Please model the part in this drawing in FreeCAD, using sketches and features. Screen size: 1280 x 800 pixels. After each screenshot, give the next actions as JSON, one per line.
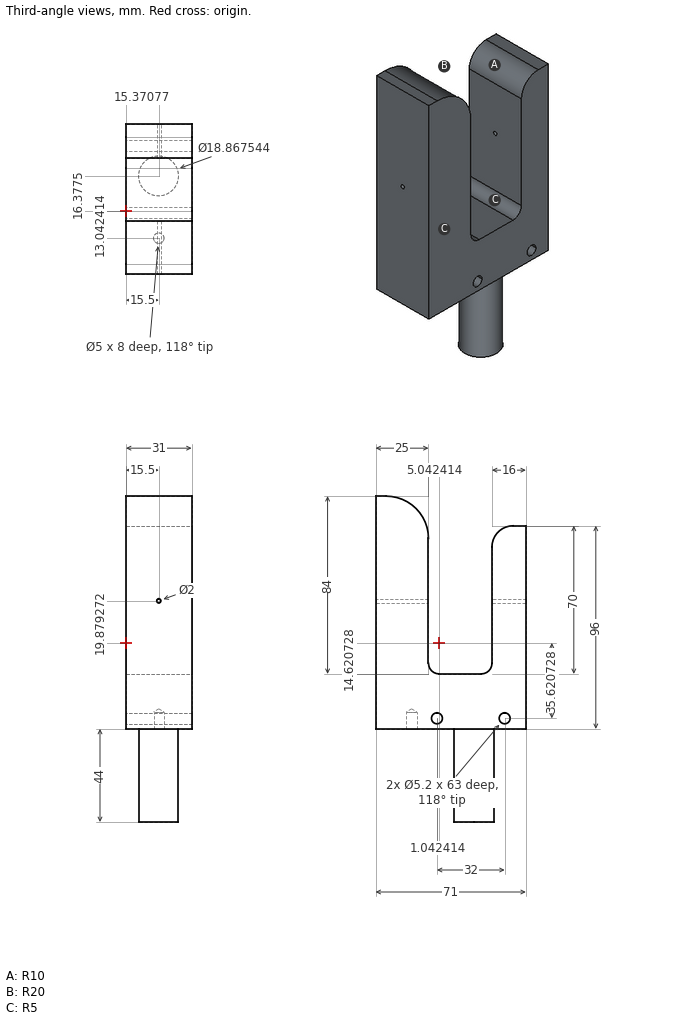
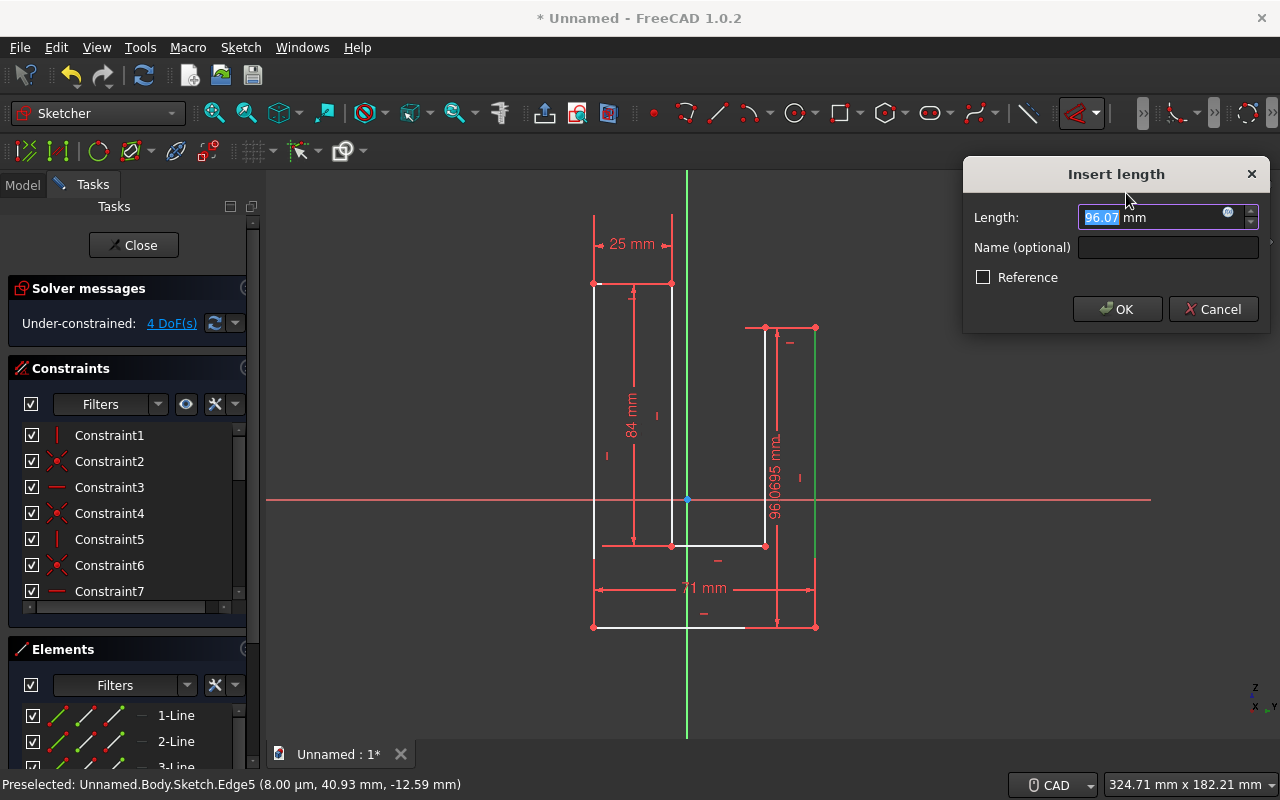
{"action": "type", "text": "96"}
{"action": "key", "text": "Return"}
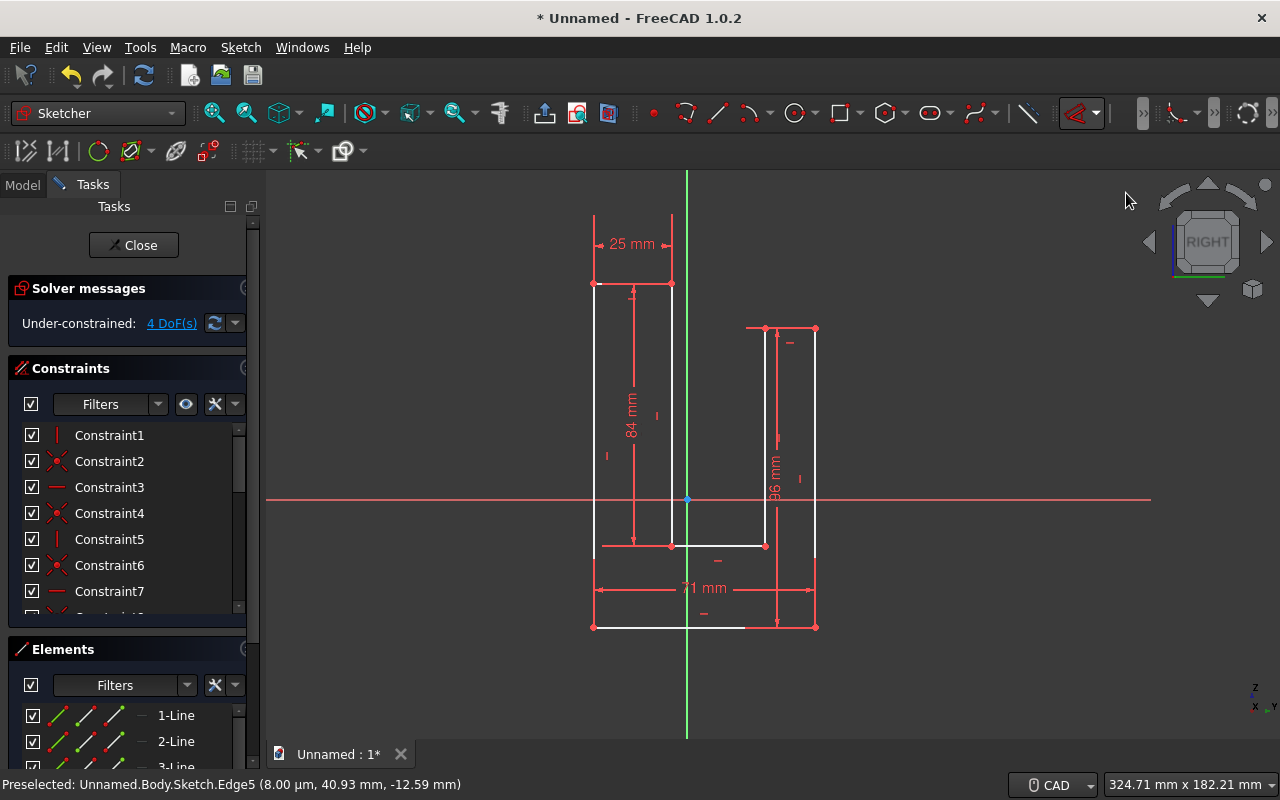
{"action": "left_click", "coordinate": [800, 328]}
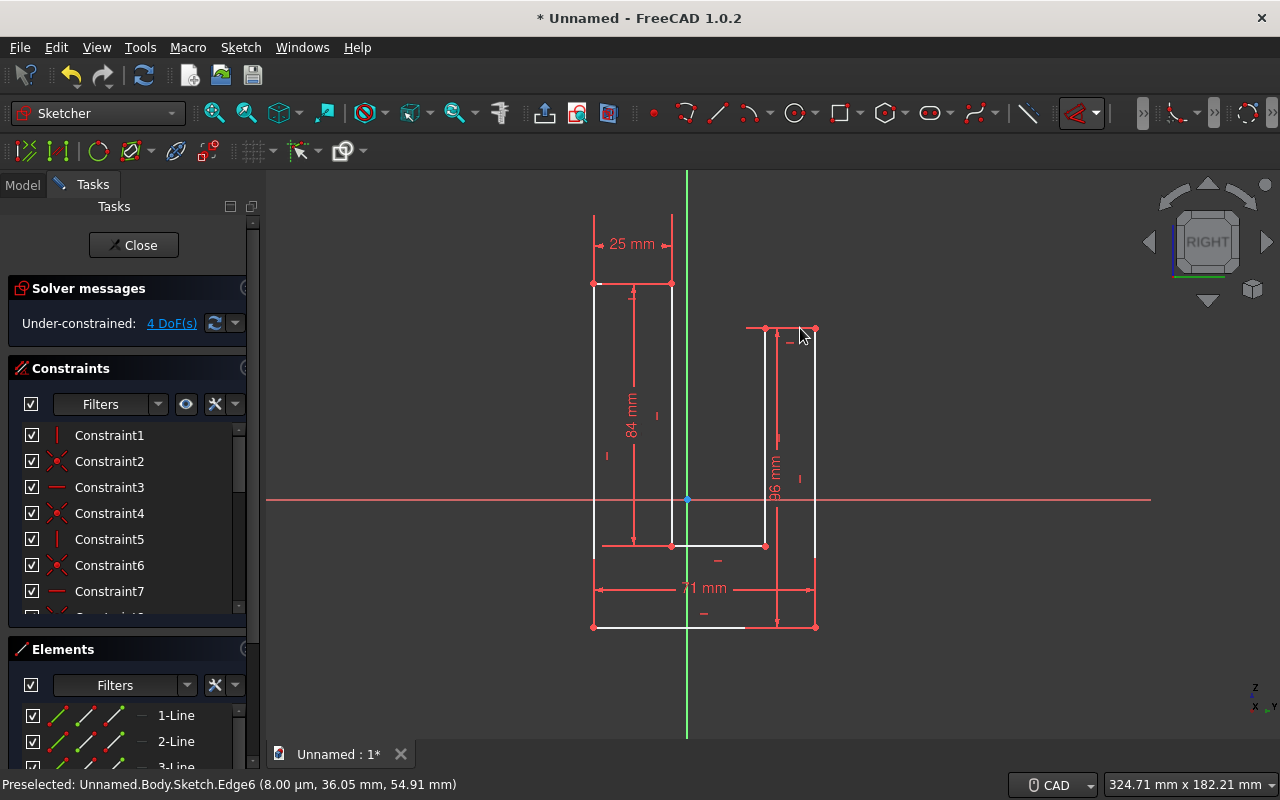
{"action": "left_click", "coordinate": [1098, 114]}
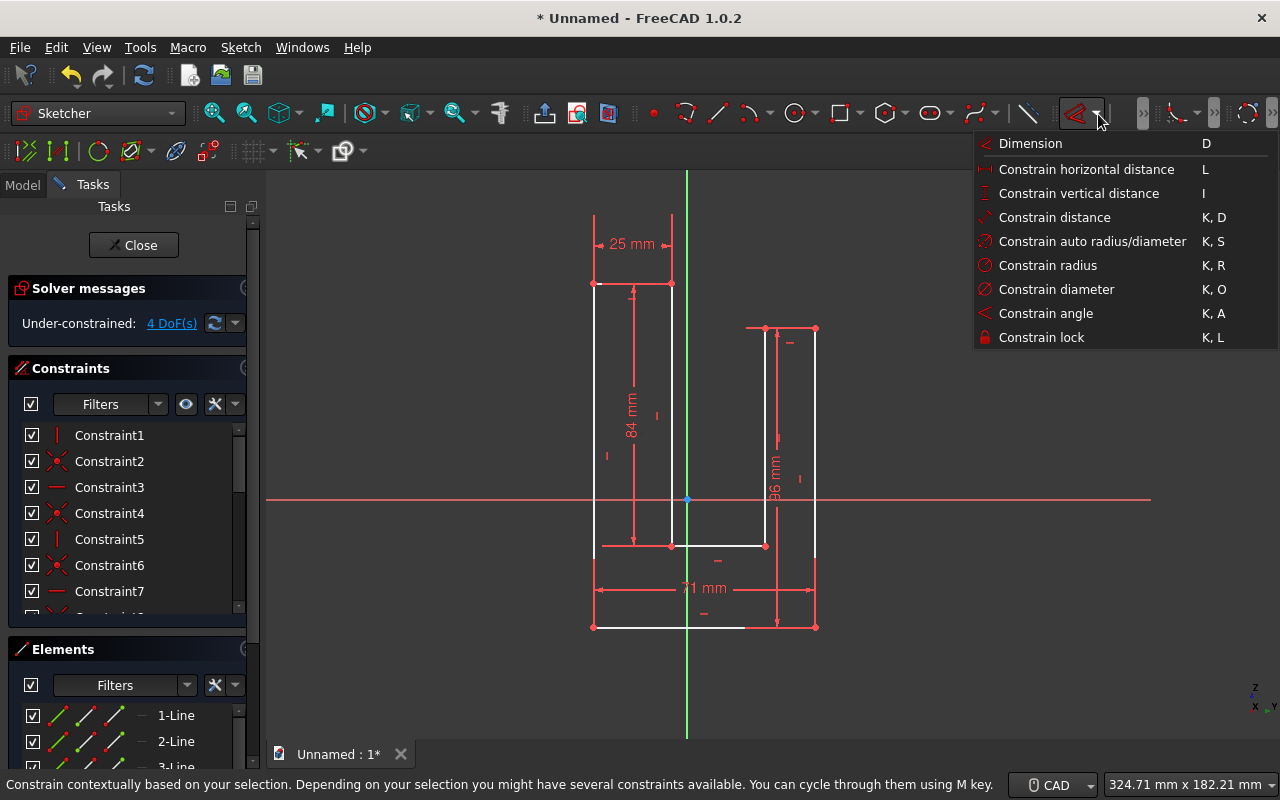
{"action": "left_click", "coordinate": [1126, 169]}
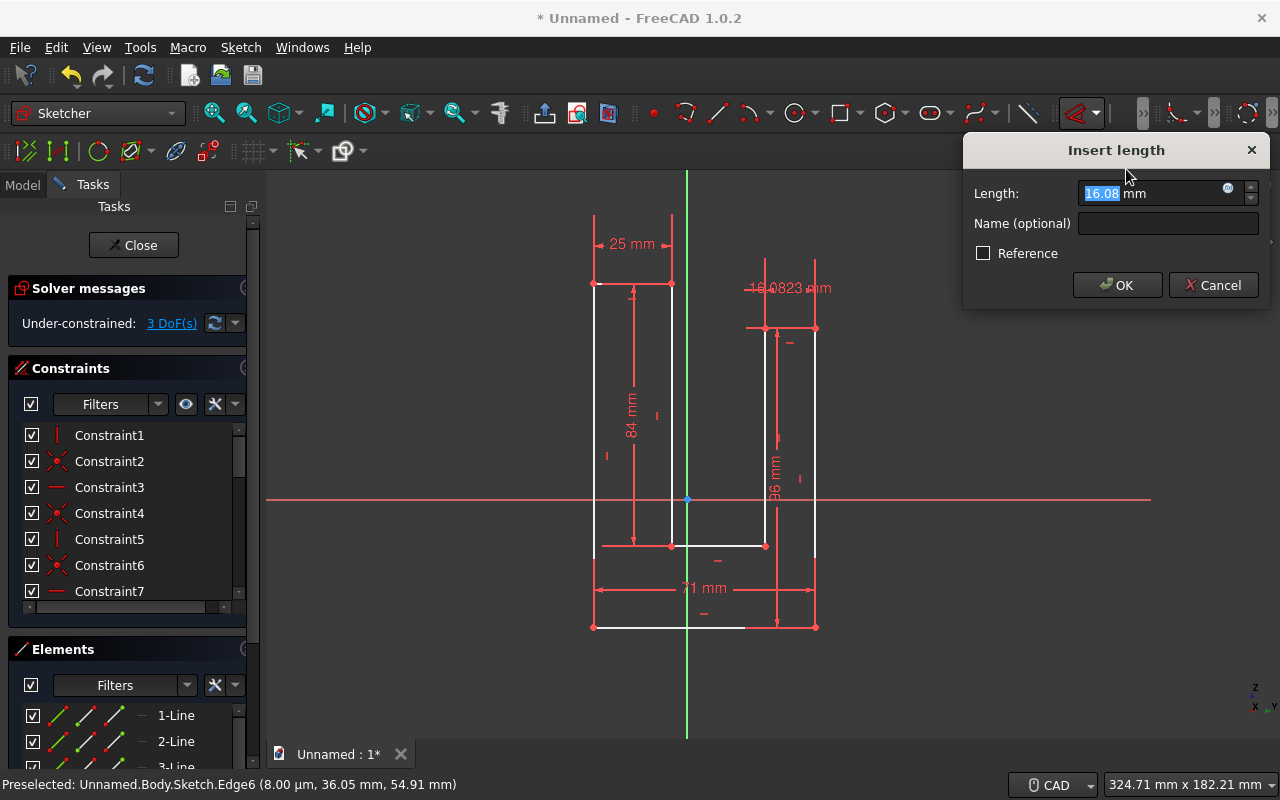
{"action": "type", "text": "16"}
{"action": "key", "text": "Return"}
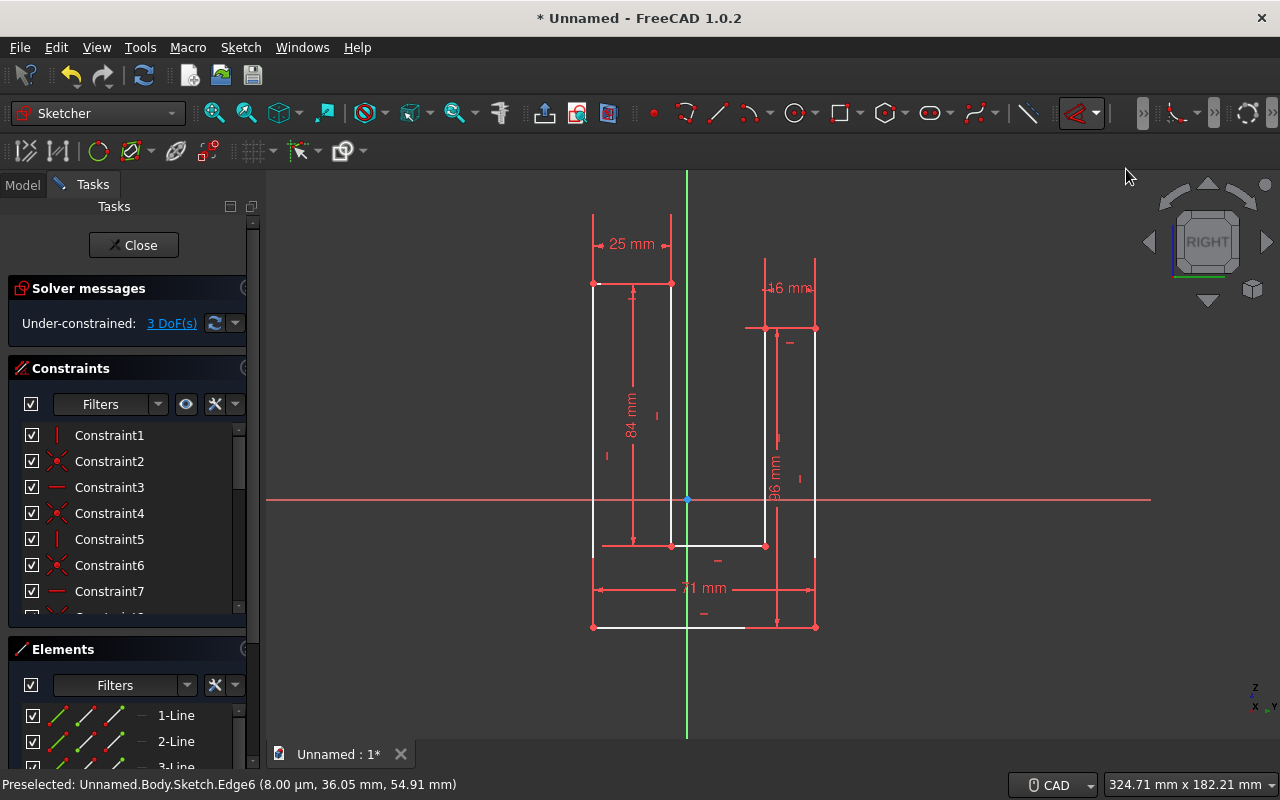
{"action": "left_click", "coordinate": [765, 394]}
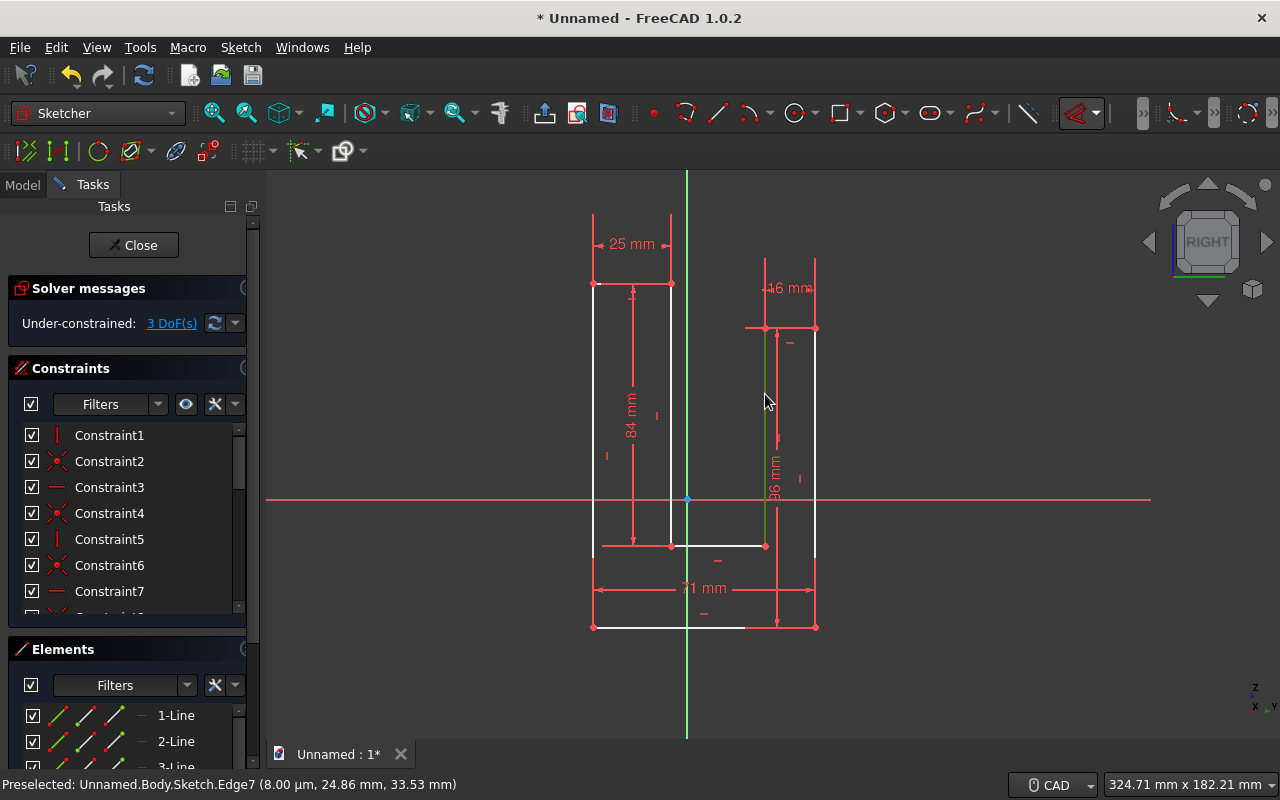
{"action": "key", "text": "i"}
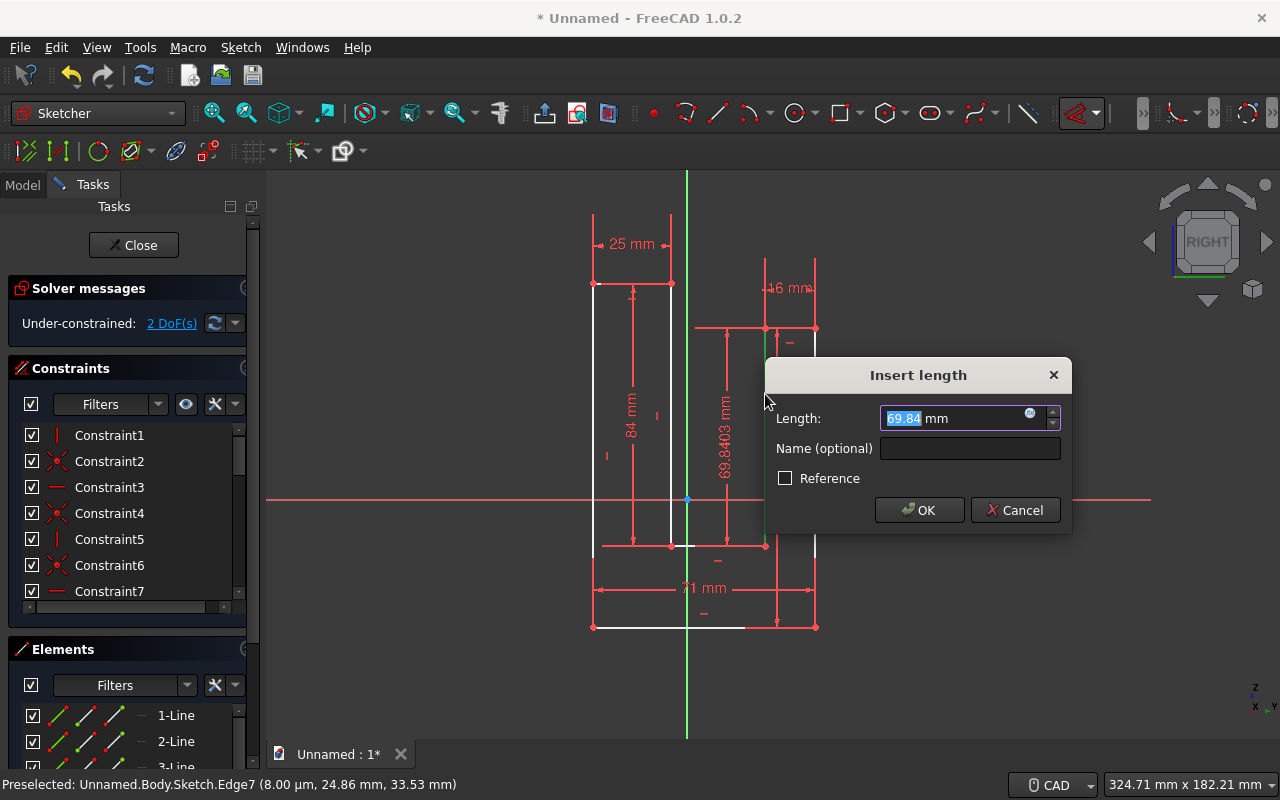
{"action": "type", "text": "70"}
{"action": "key", "text": "Return"}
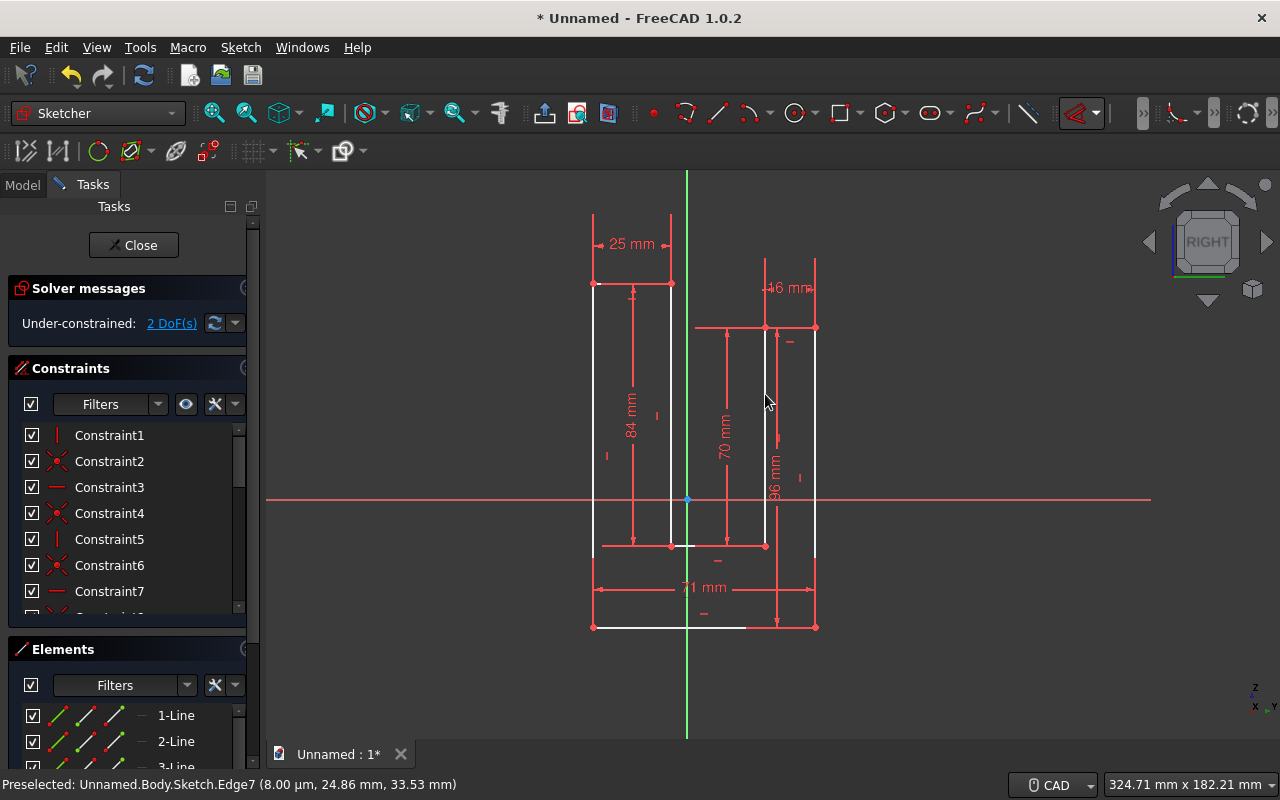
{"action": "scroll", "coordinate": [671, 546], "scroll_direction": "up", "scroll_amount": 5}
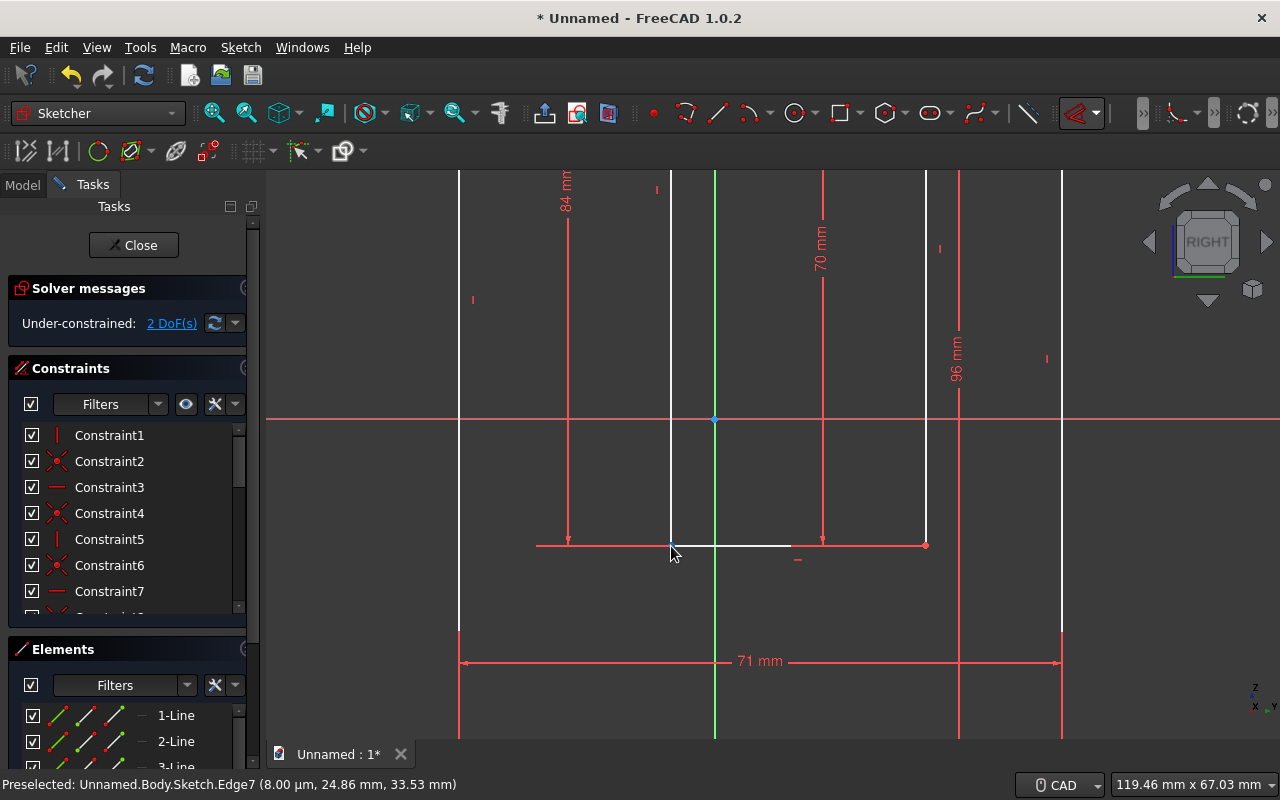
{"action": "left_click", "coordinate": [671, 546]}